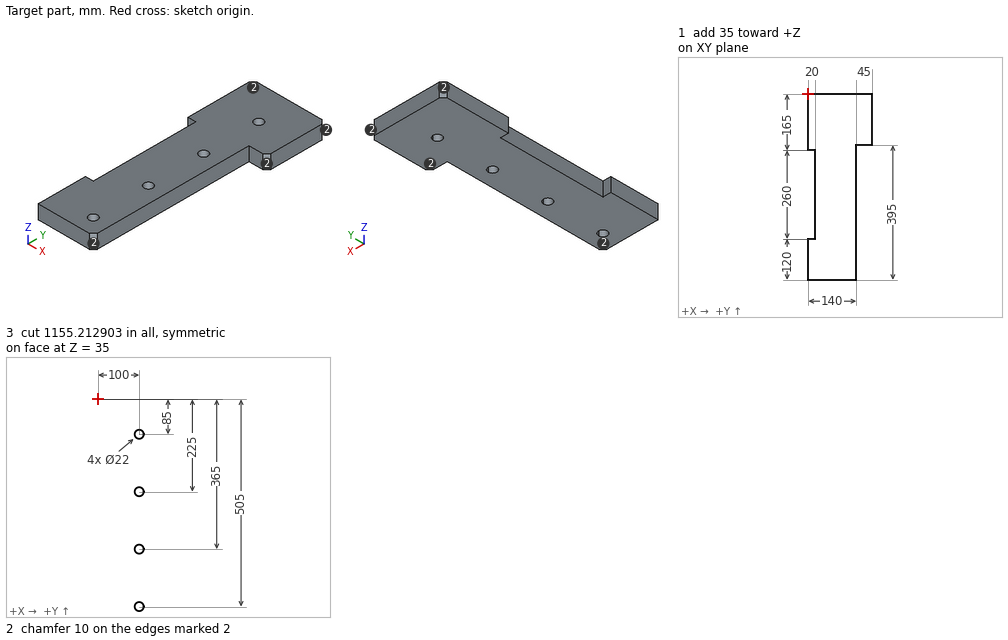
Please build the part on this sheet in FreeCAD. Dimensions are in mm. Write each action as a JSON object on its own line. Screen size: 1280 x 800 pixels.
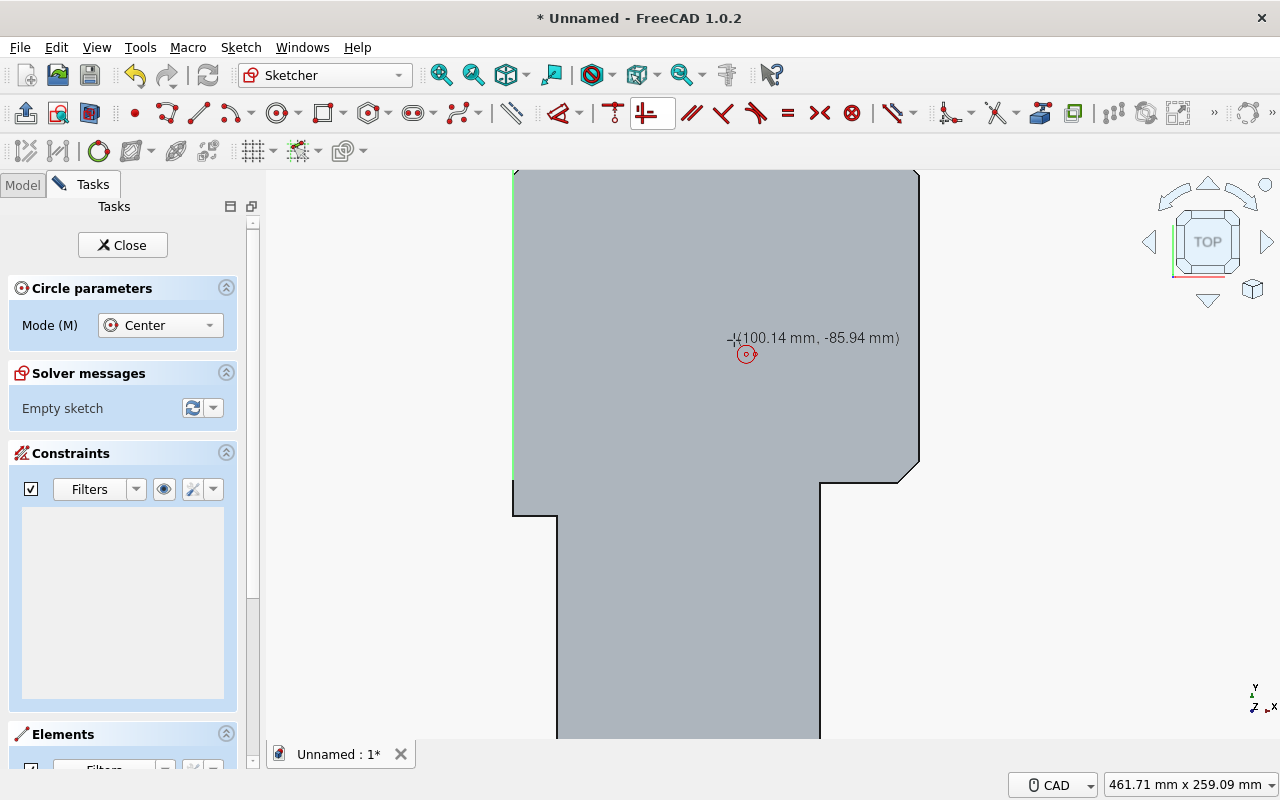
{"action": "left_click", "coordinate": [733, 341]}
{"action": "mouse_move", "coordinate": [750, 323]}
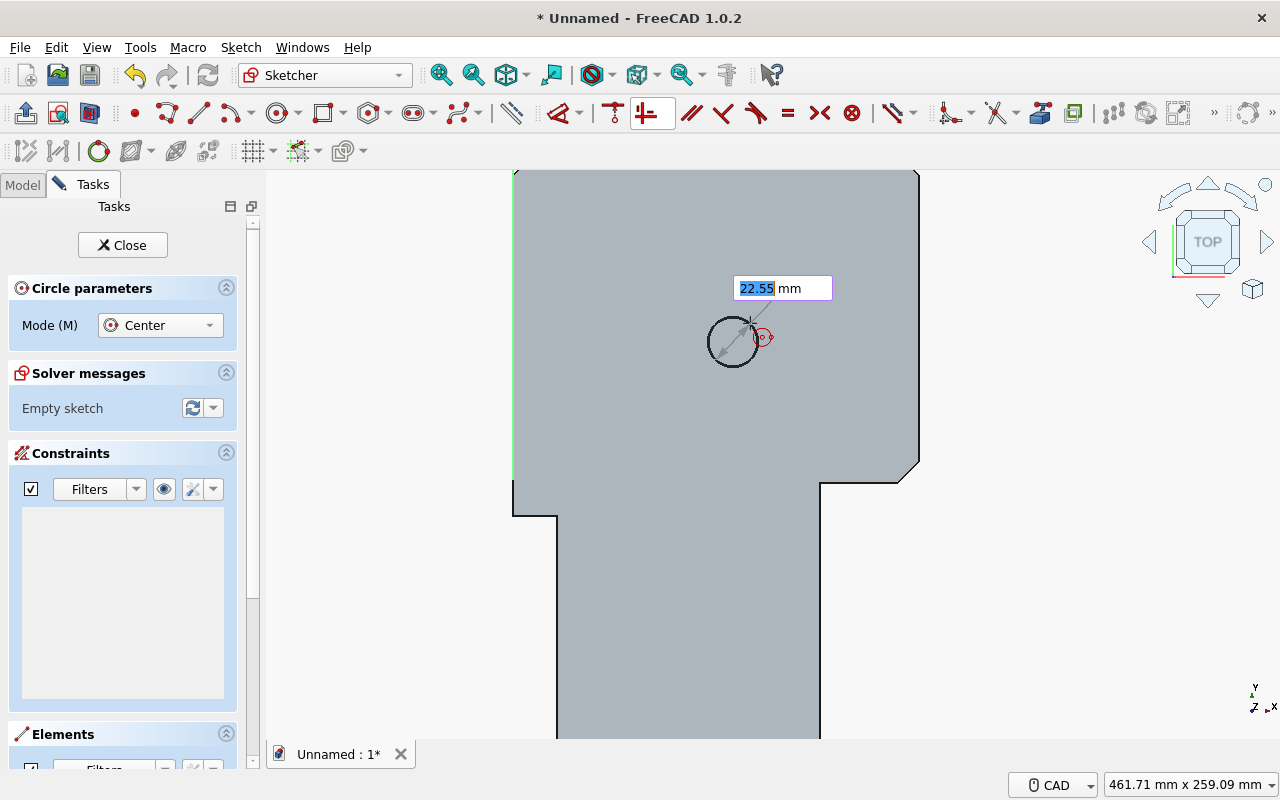
{"action": "type", "text": "22"}
{"action": "key", "text": "Return"}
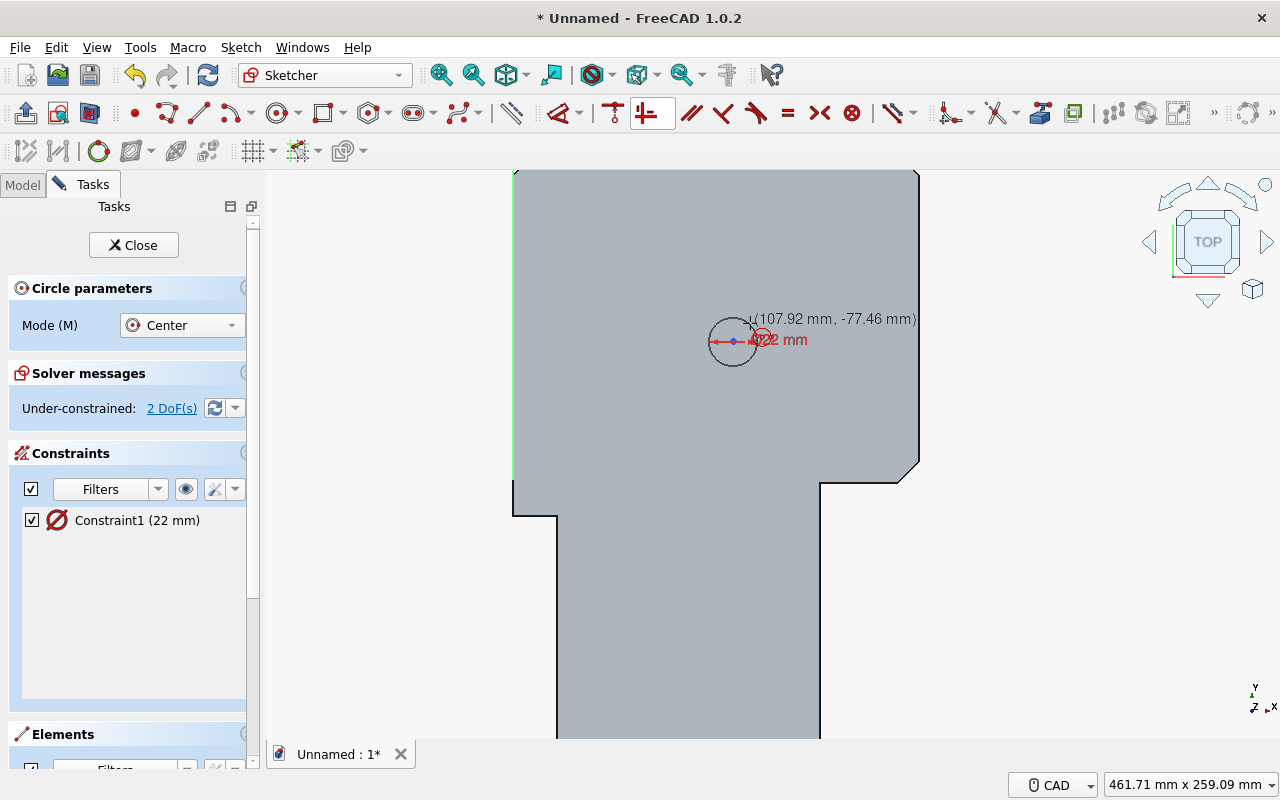
{"action": "left_click", "coordinate": [733, 648]}
{"action": "mouse_move", "coordinate": [750, 631]}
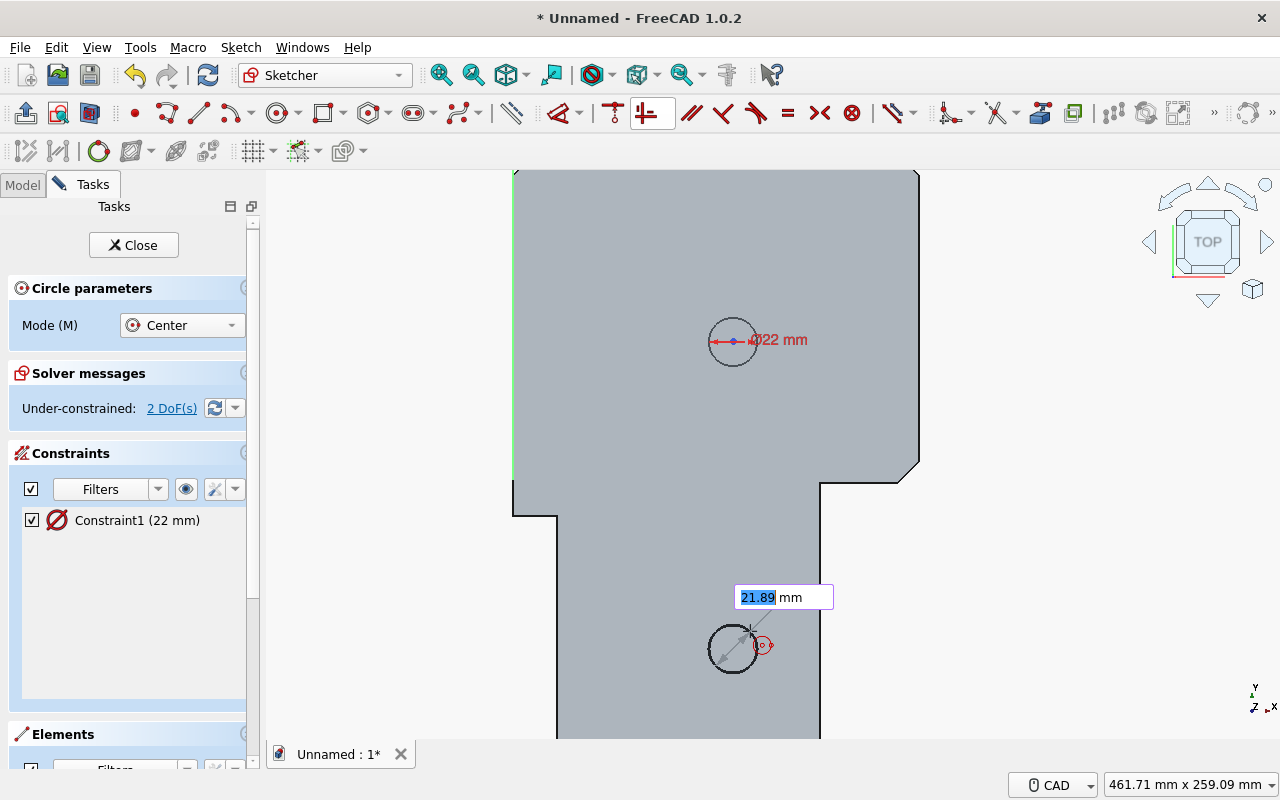
{"action": "type", "text": "22"}
{"action": "key", "text": "Return"}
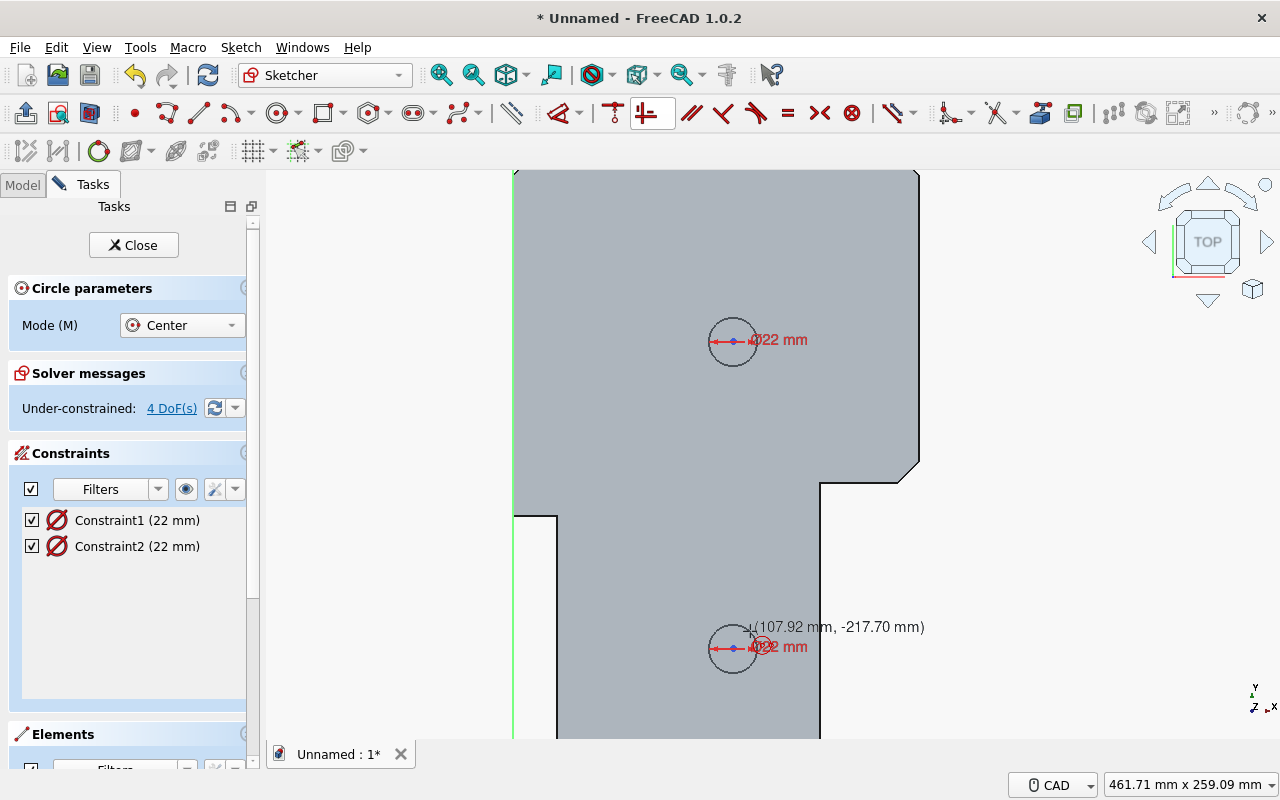
{"action": "scroll", "coordinate": [735, 340], "scroll_direction": "down", "scroll_amount": 6}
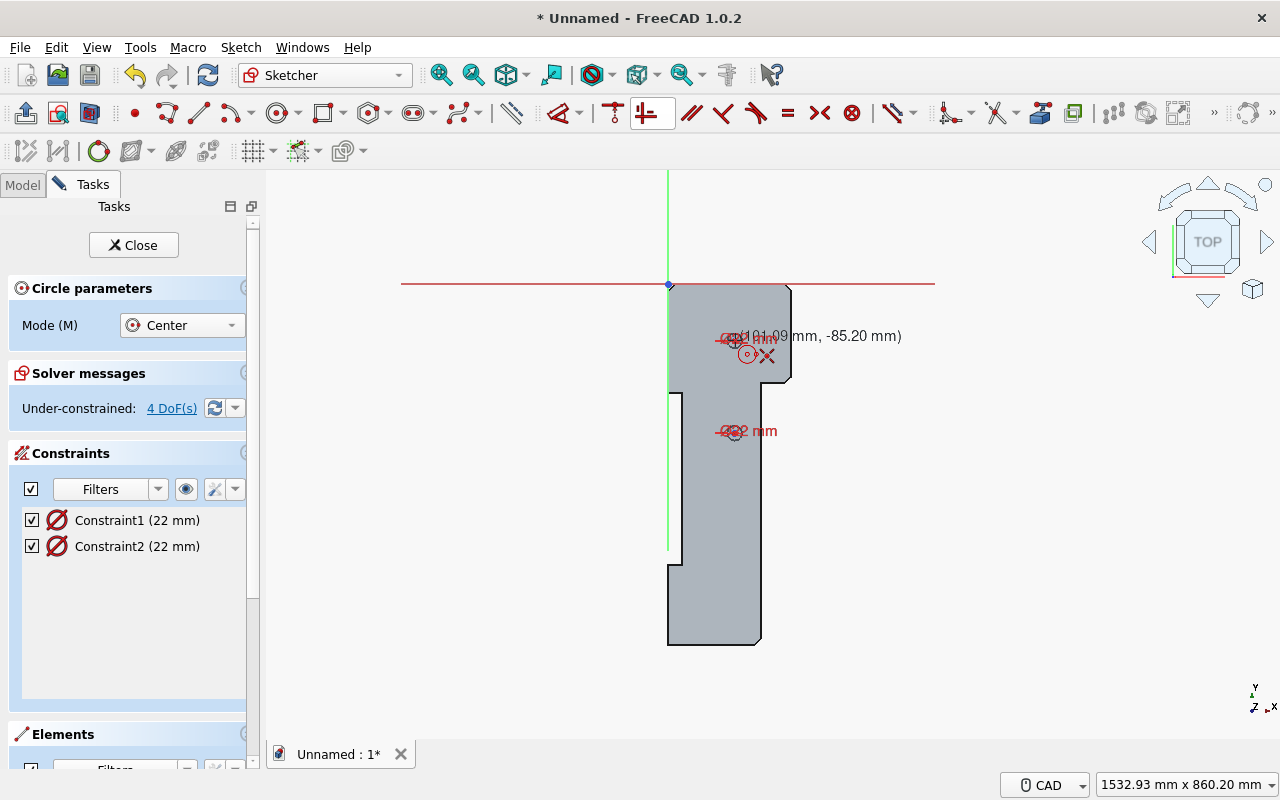
{"action": "scroll", "coordinate": [735, 526], "scroll_direction": "up", "scroll_amount": 6}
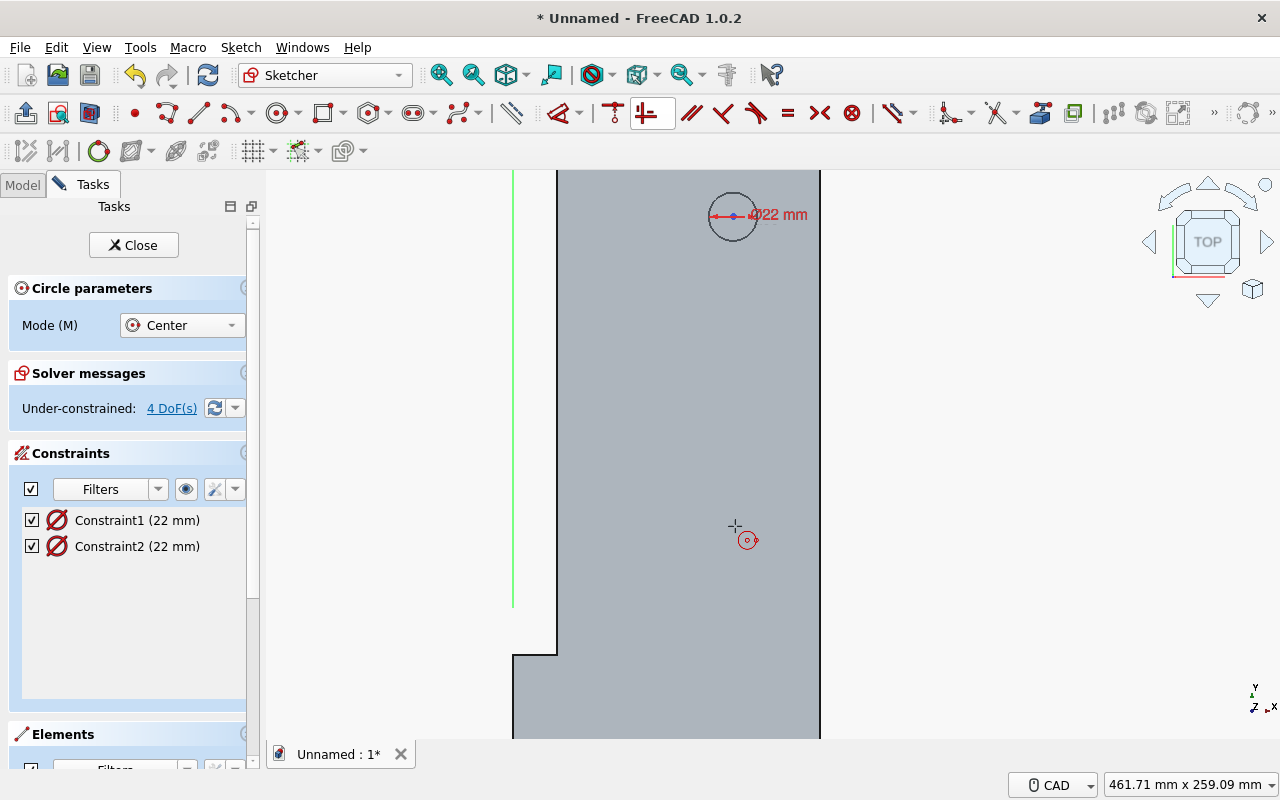
{"action": "left_click", "coordinate": [733, 523]}
{"action": "mouse_move", "coordinate": [750, 506]}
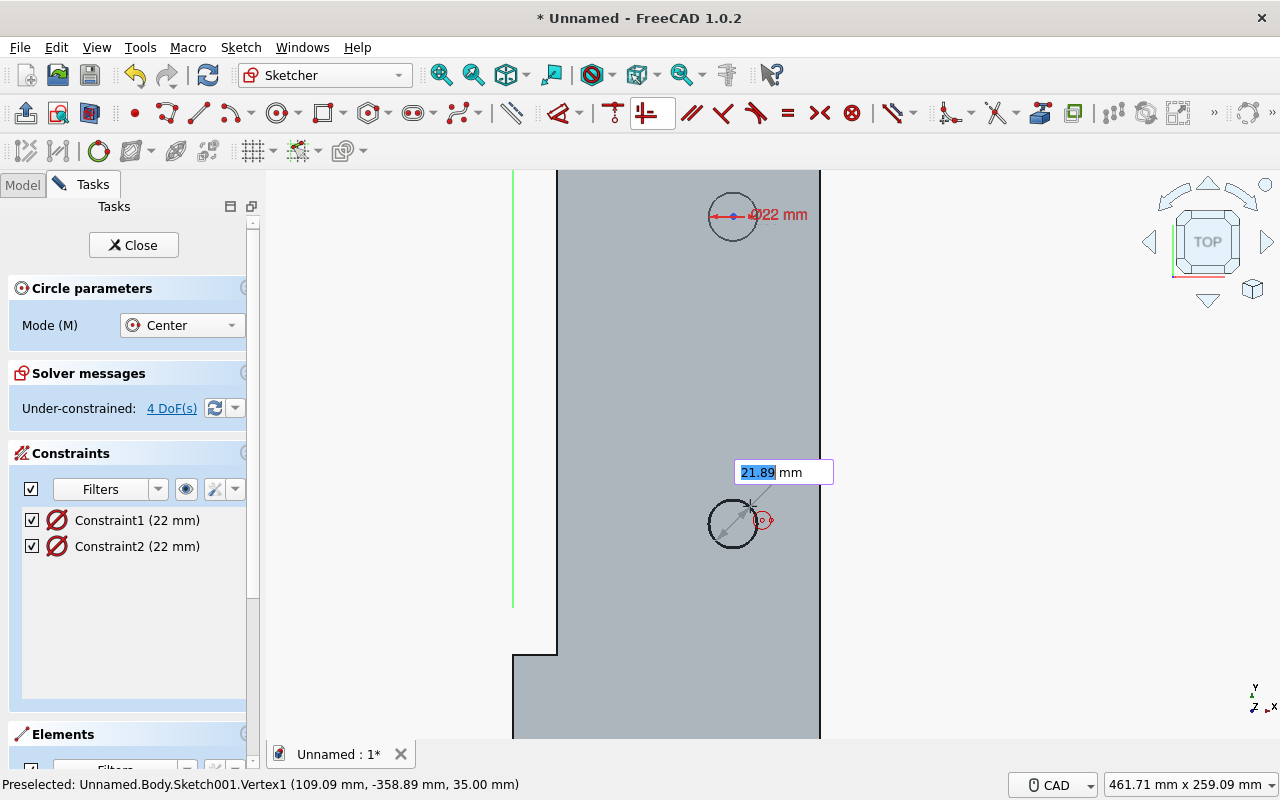
{"action": "type", "text": "22"}
{"action": "key", "text": "Return"}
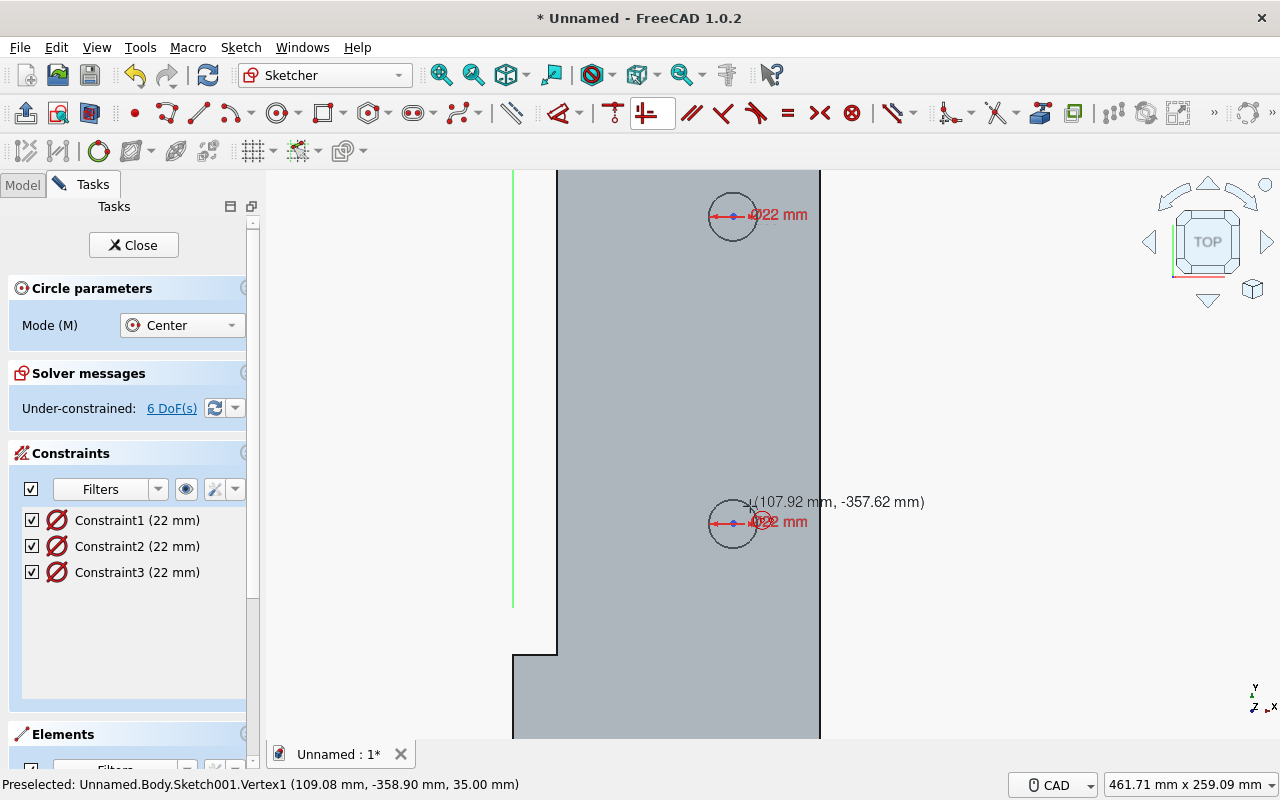
{"action": "scroll", "coordinate": [735, 526], "scroll_direction": "down", "scroll_amount": 6}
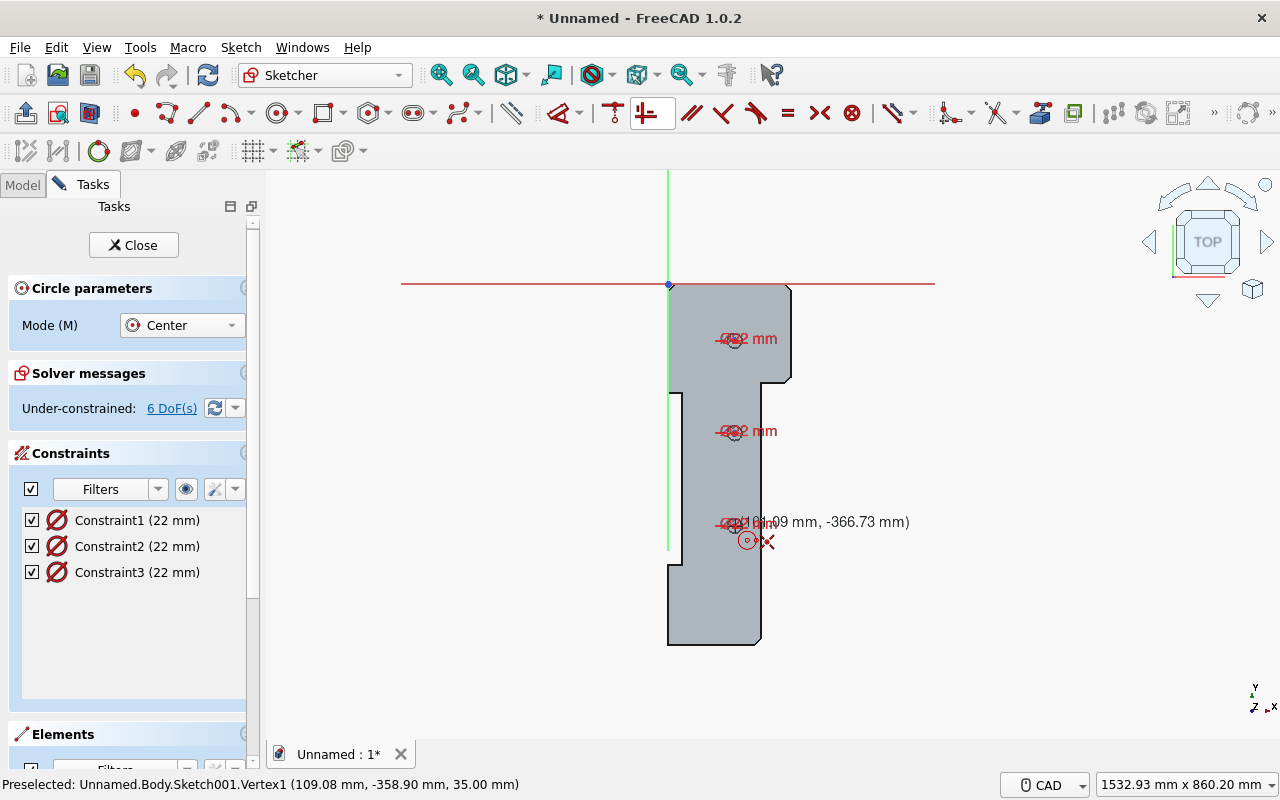
{"action": "scroll", "coordinate": [735, 618], "scroll_direction": "up", "scroll_amount": 6}